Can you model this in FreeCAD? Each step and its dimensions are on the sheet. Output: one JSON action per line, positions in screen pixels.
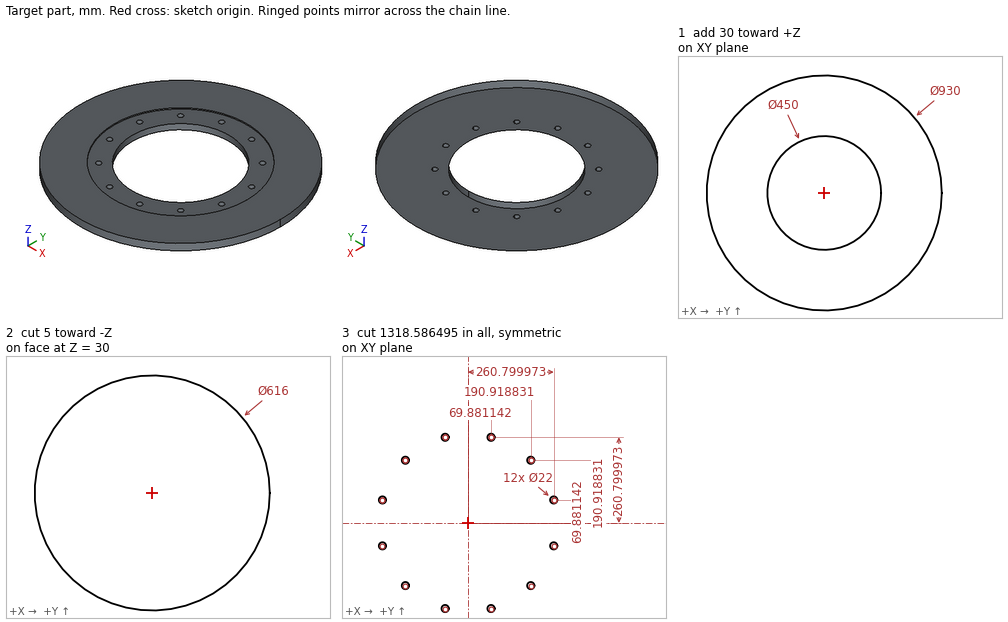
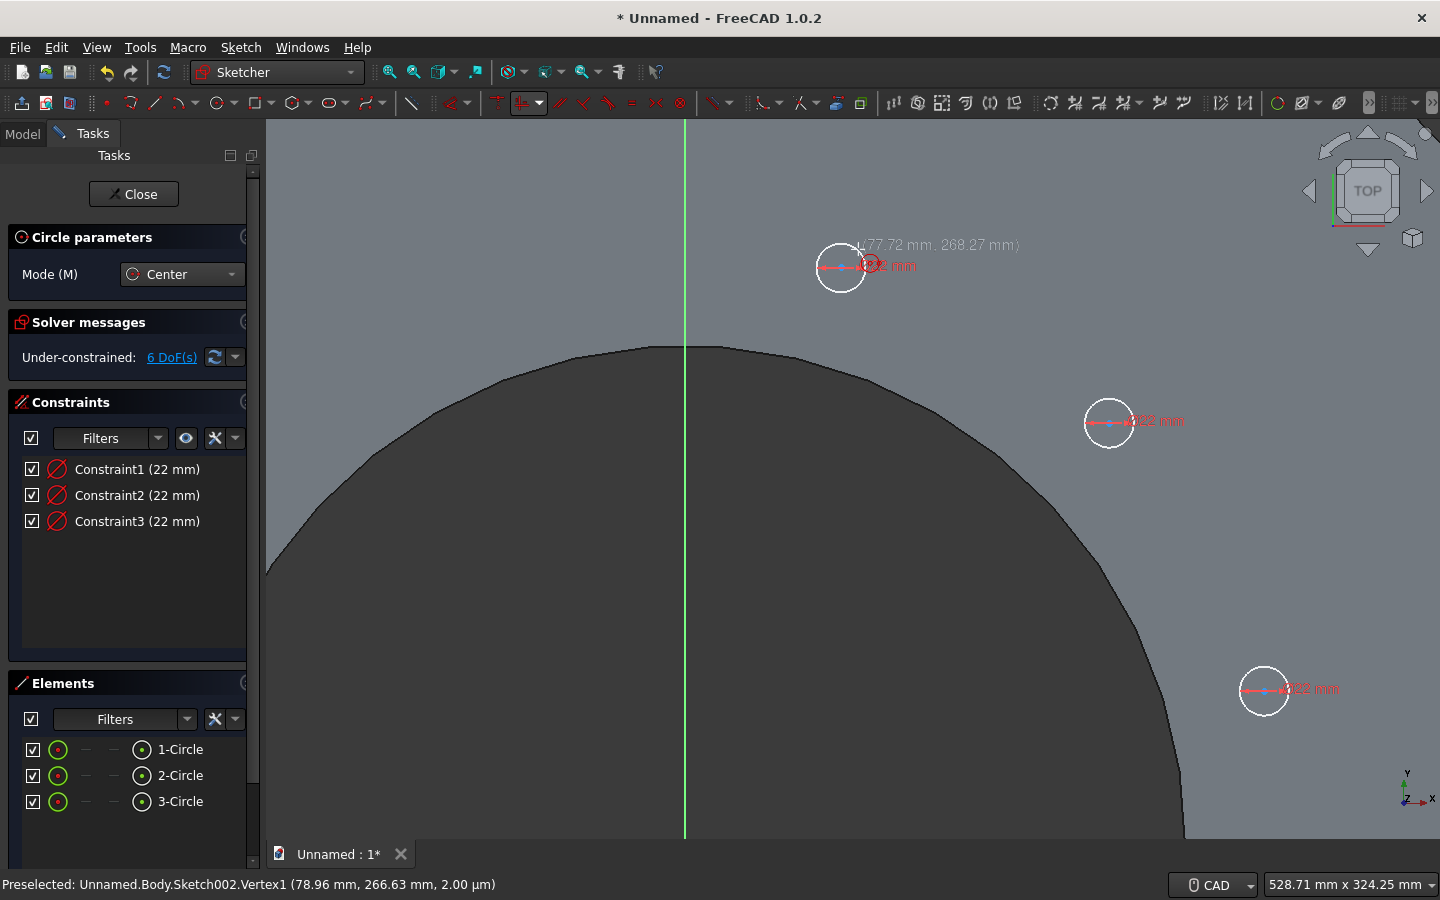
{"action": "left_click", "coordinate": [530, 267]}
{"action": "mouse_move", "coordinate": [548, 249]}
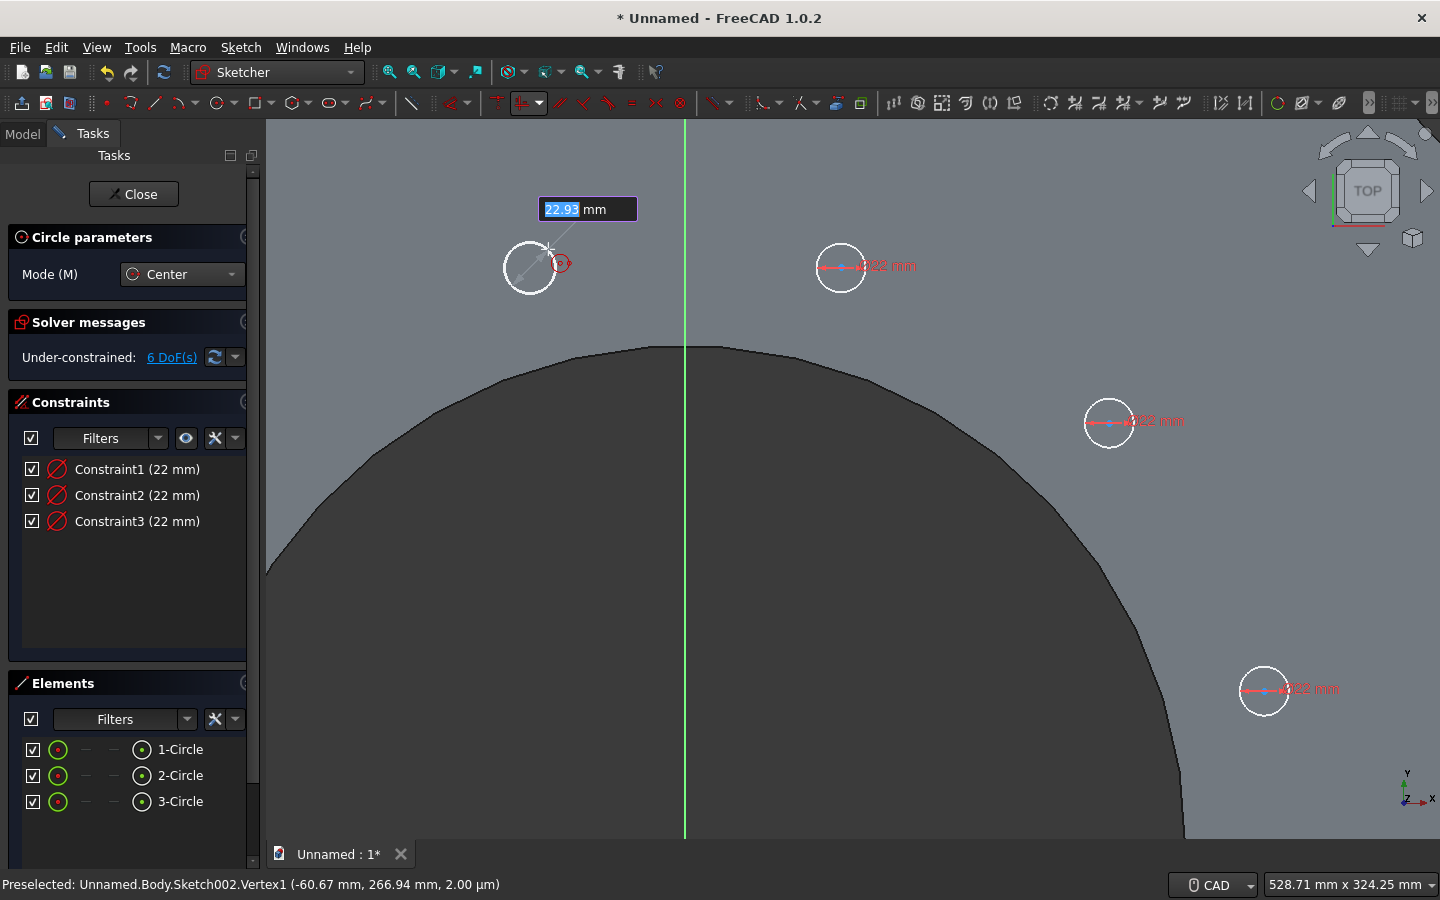
{"action": "type", "text": "22"}
{"action": "key", "text": "Return"}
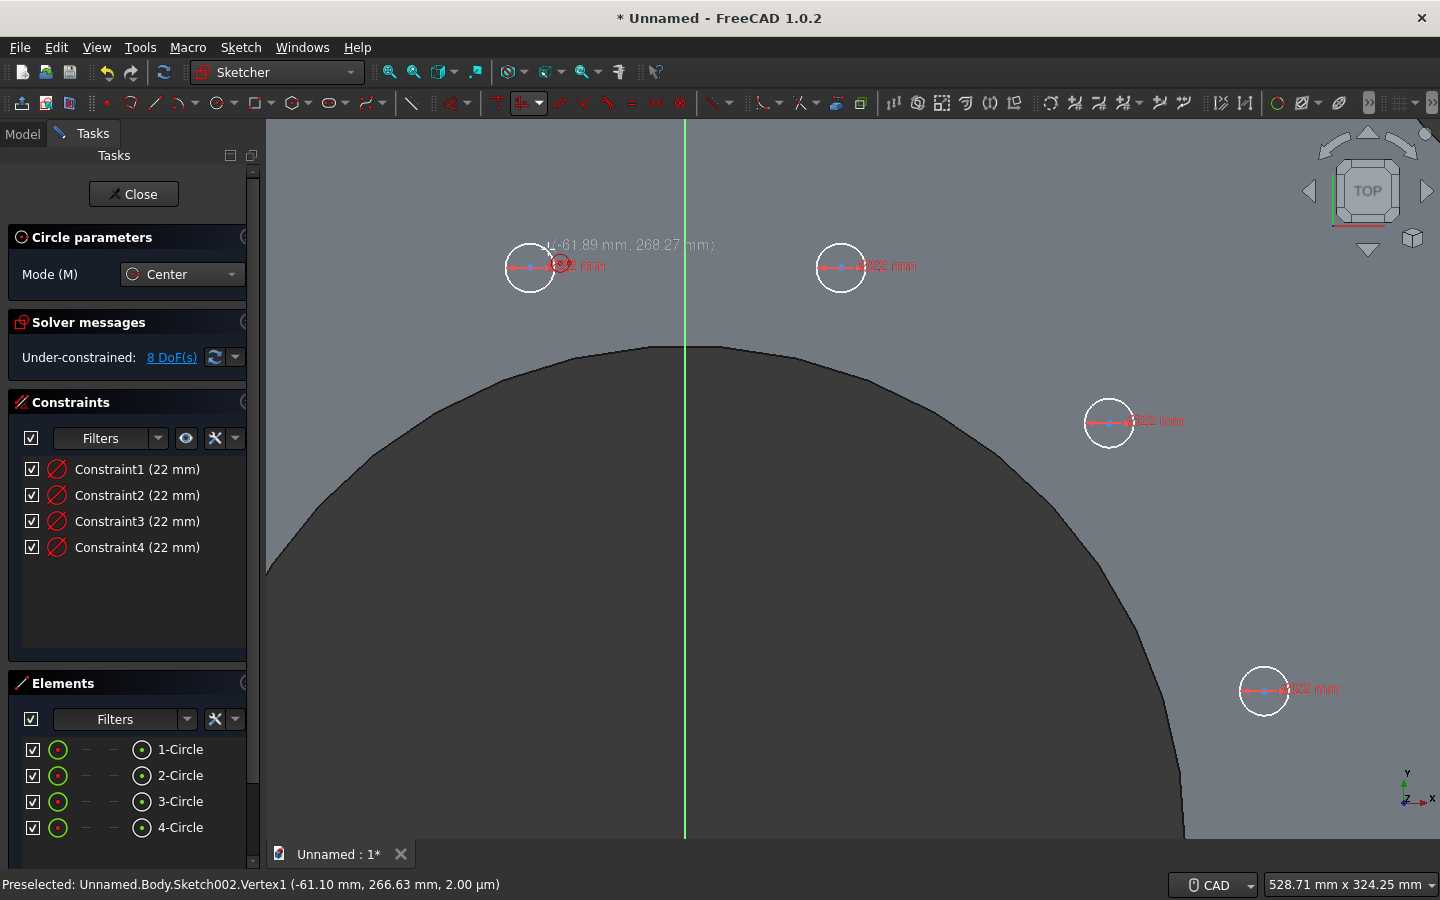
{"action": "scroll", "coordinate": [842, 266], "scroll_direction": "down", "scroll_amount": 5}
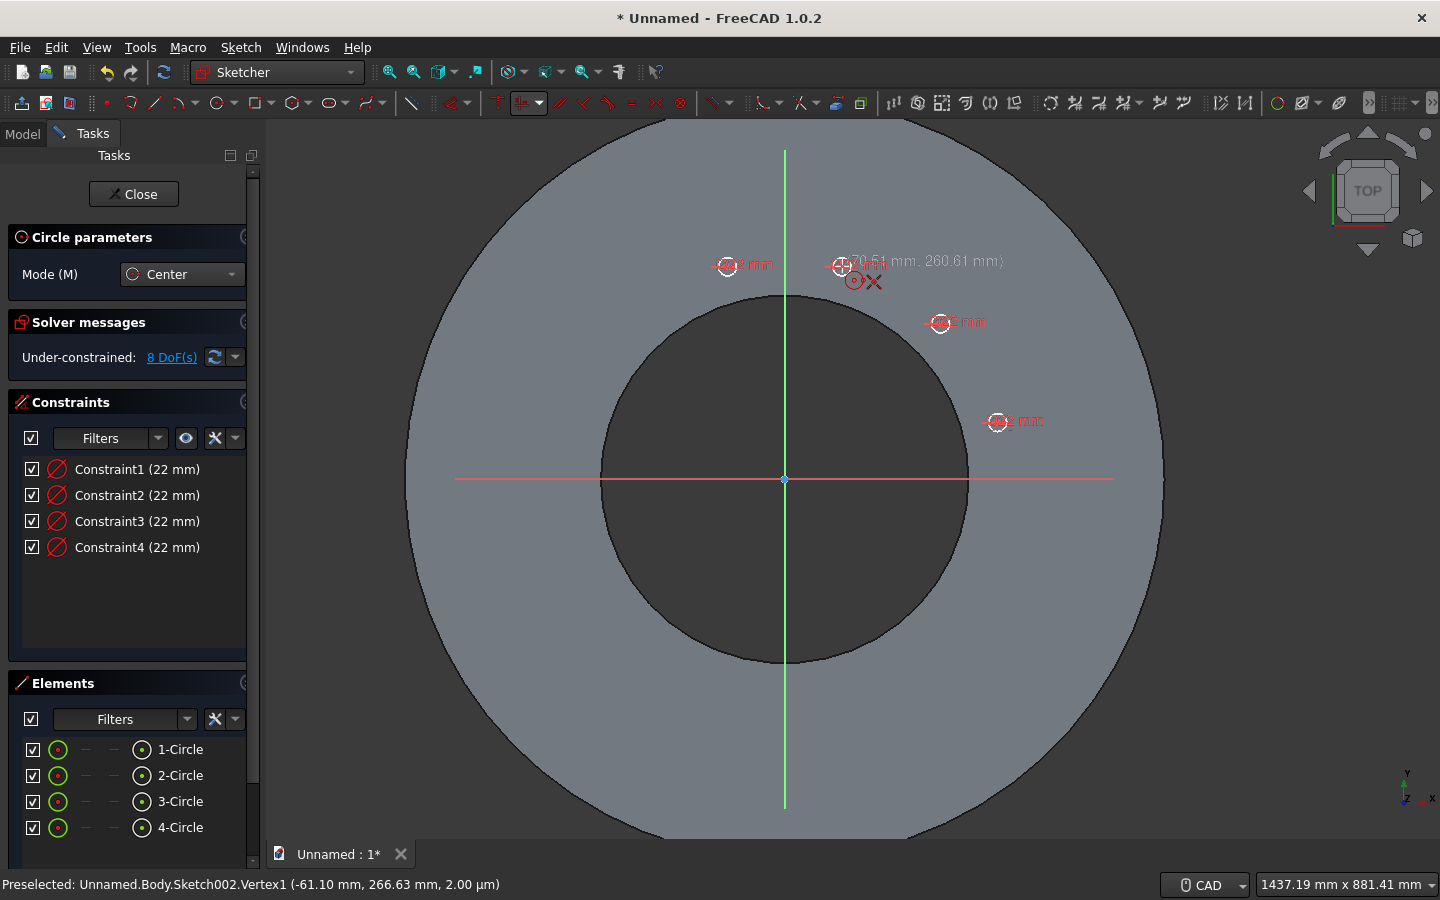
{"action": "scroll", "coordinate": [629, 323], "scroll_direction": "up", "scroll_amount": 5}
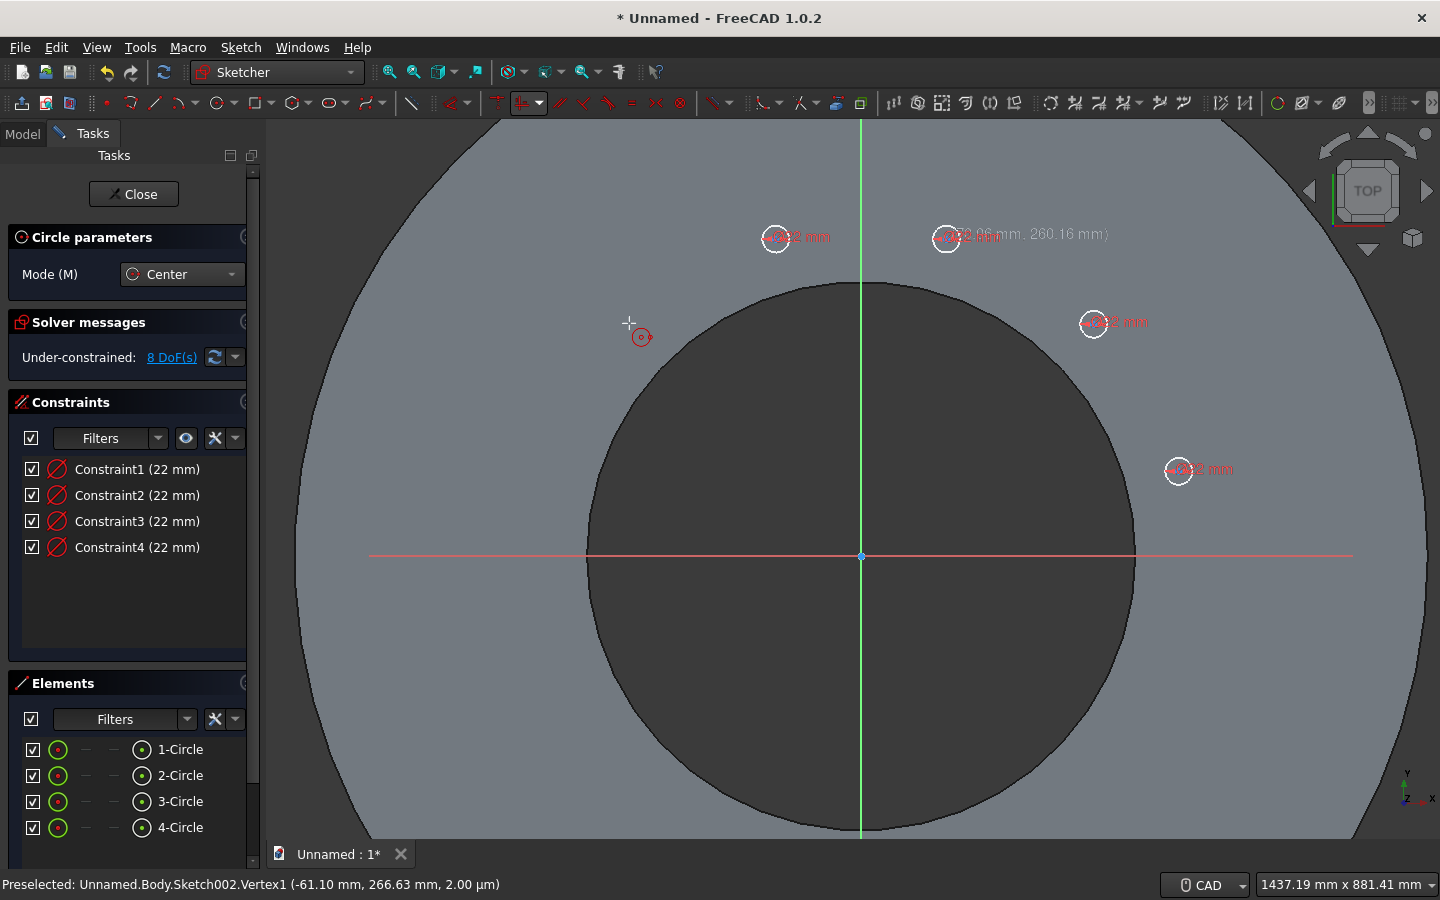
{"action": "left_click", "coordinate": [628, 324]}
{"action": "mouse_move", "coordinate": [645, 306]}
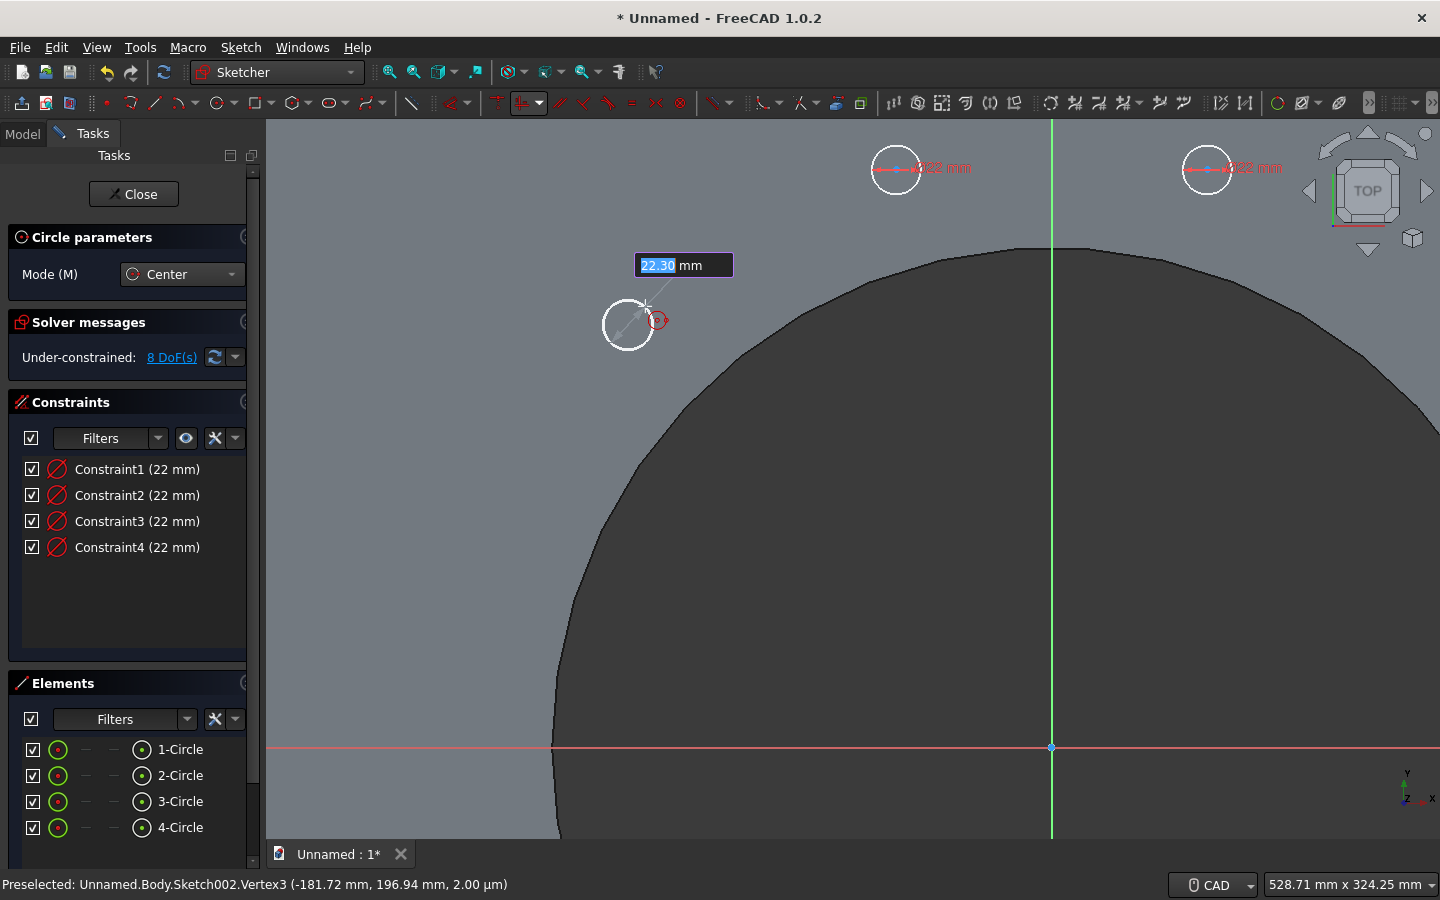
{"action": "type", "text": "22"}
{"action": "key", "text": "Return"}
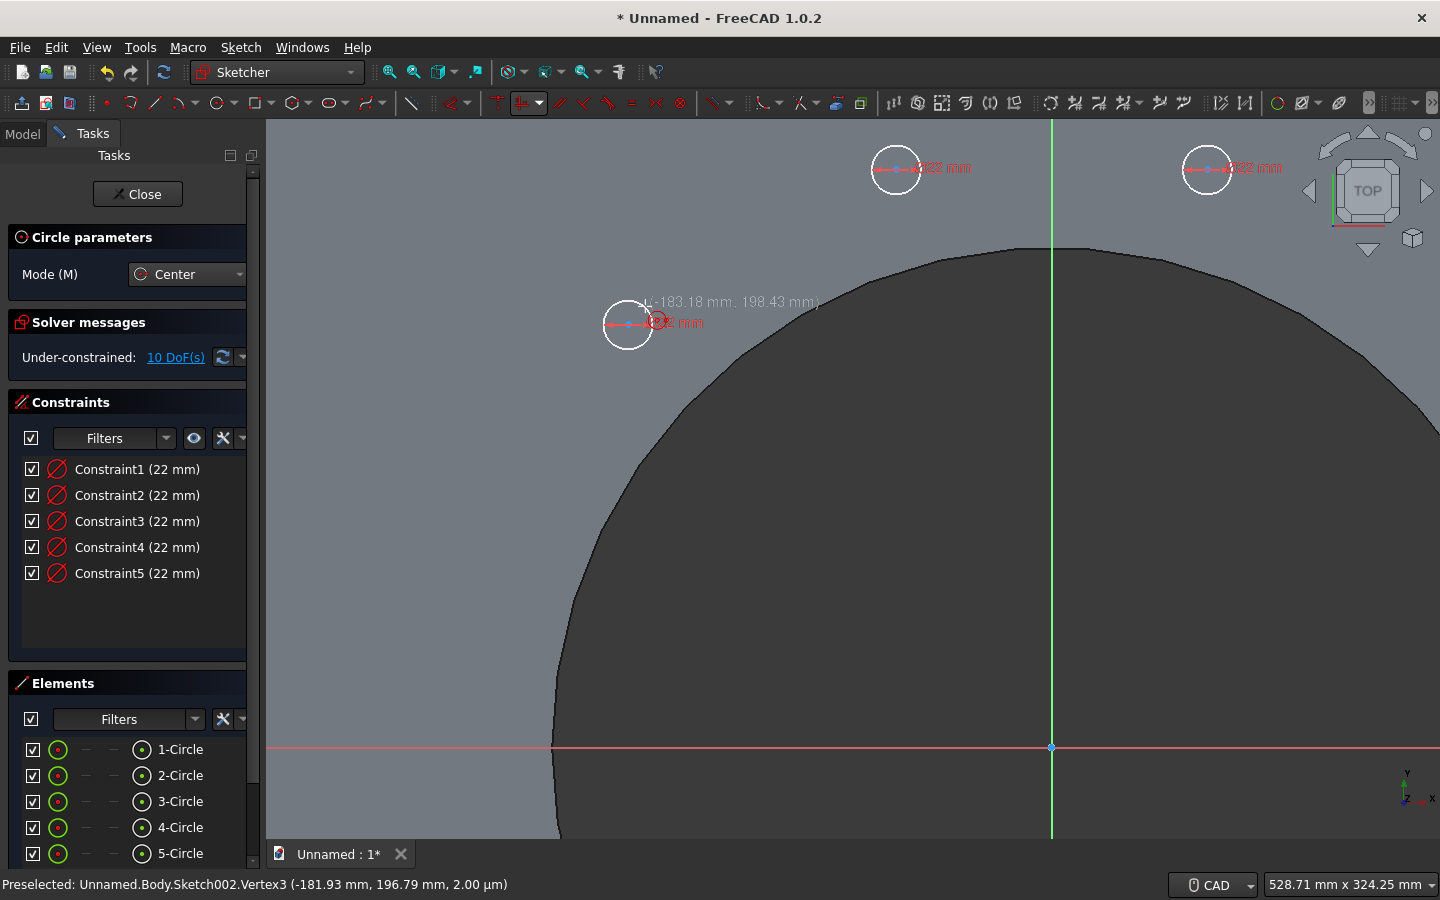
{"action": "left_click", "coordinate": [473, 592]}
{"action": "mouse_move", "coordinate": [490, 575]}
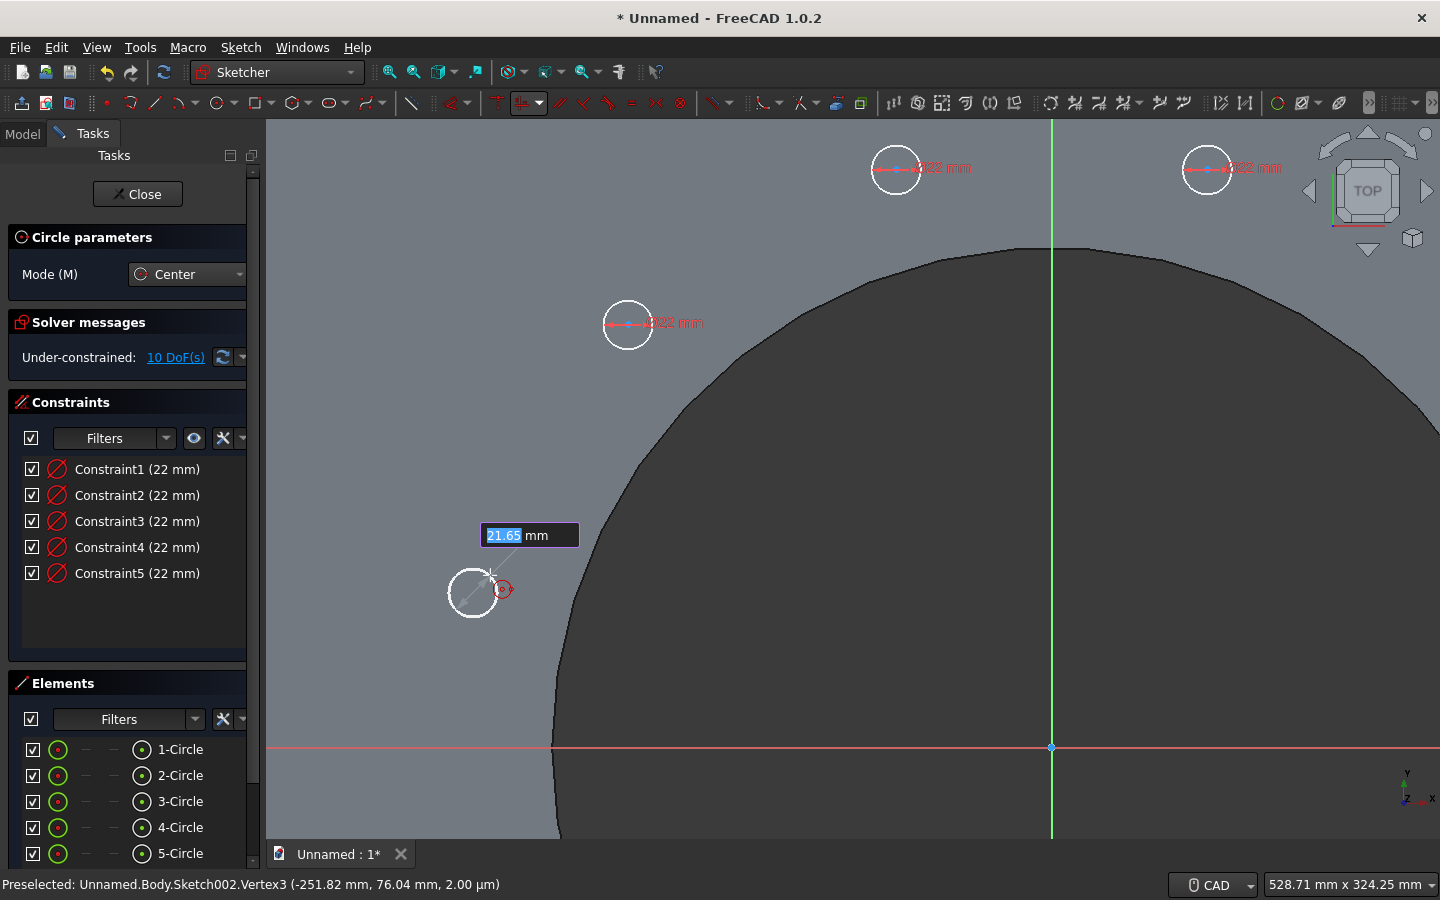
{"action": "type", "text": "22"}
{"action": "key", "text": "Return"}